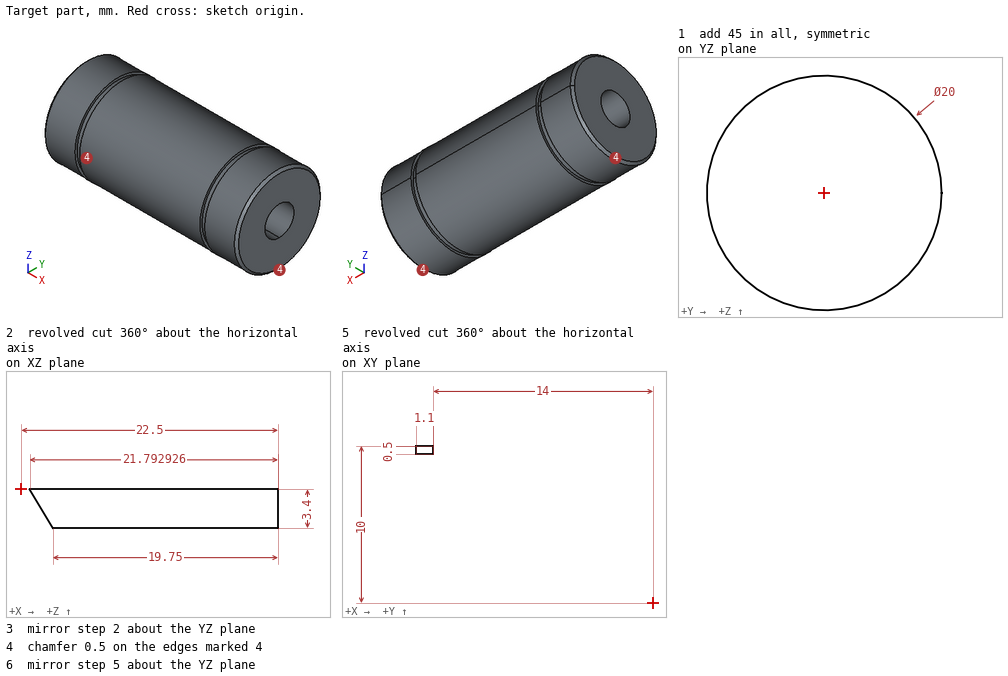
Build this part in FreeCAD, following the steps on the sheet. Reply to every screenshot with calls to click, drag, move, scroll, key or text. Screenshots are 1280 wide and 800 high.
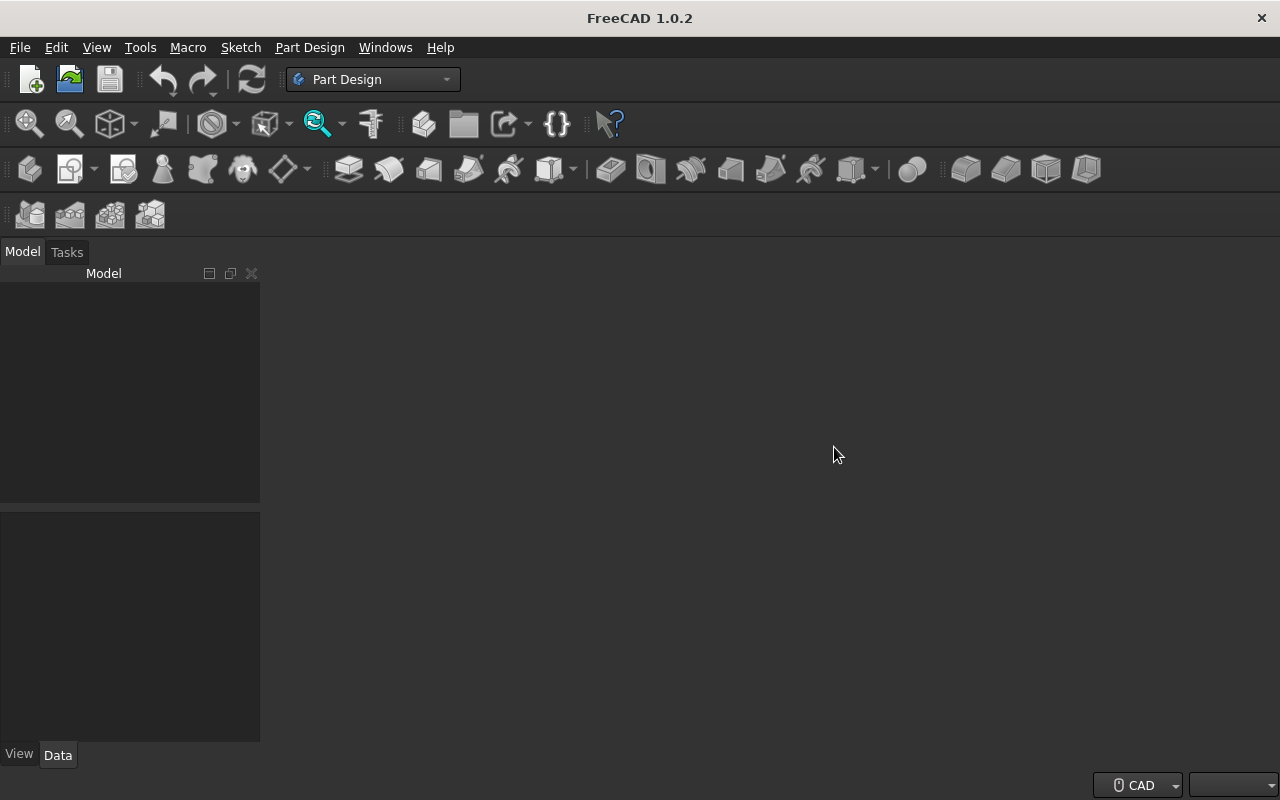
click(30, 80)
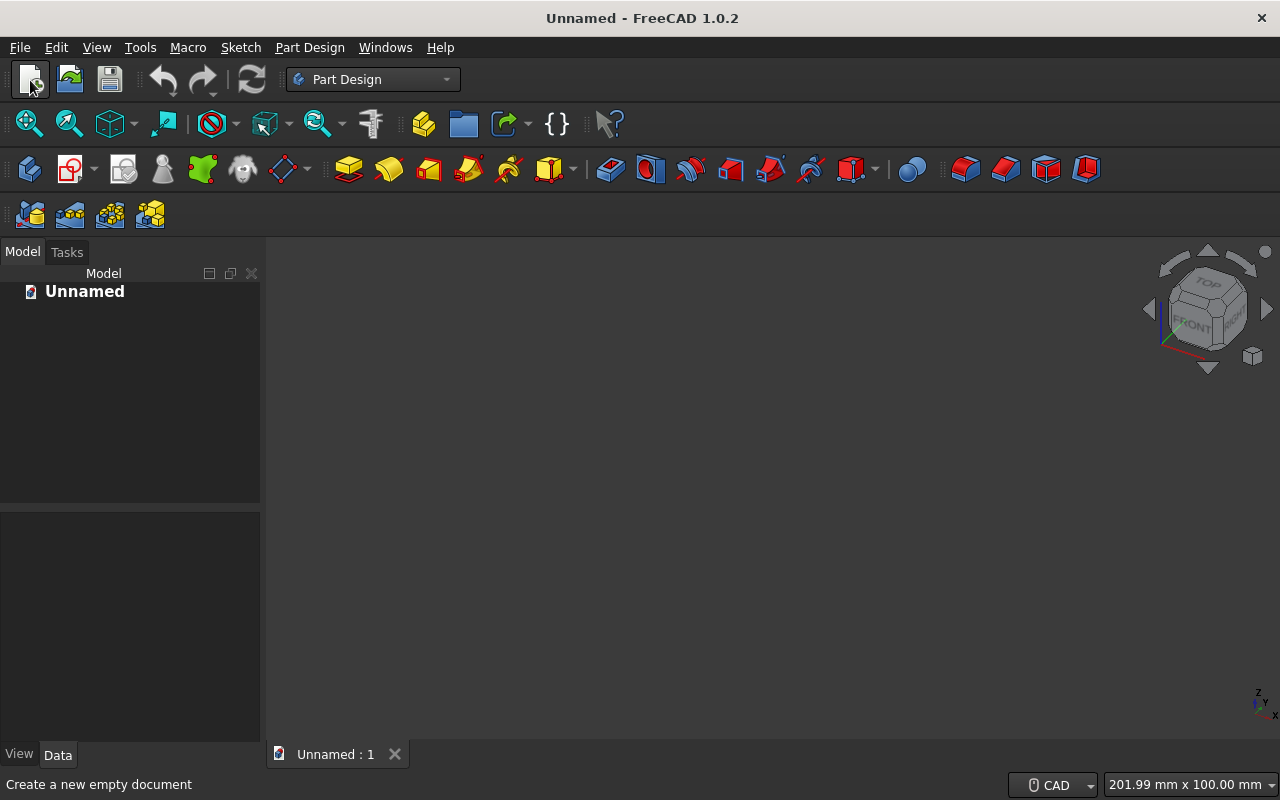
click(70, 170)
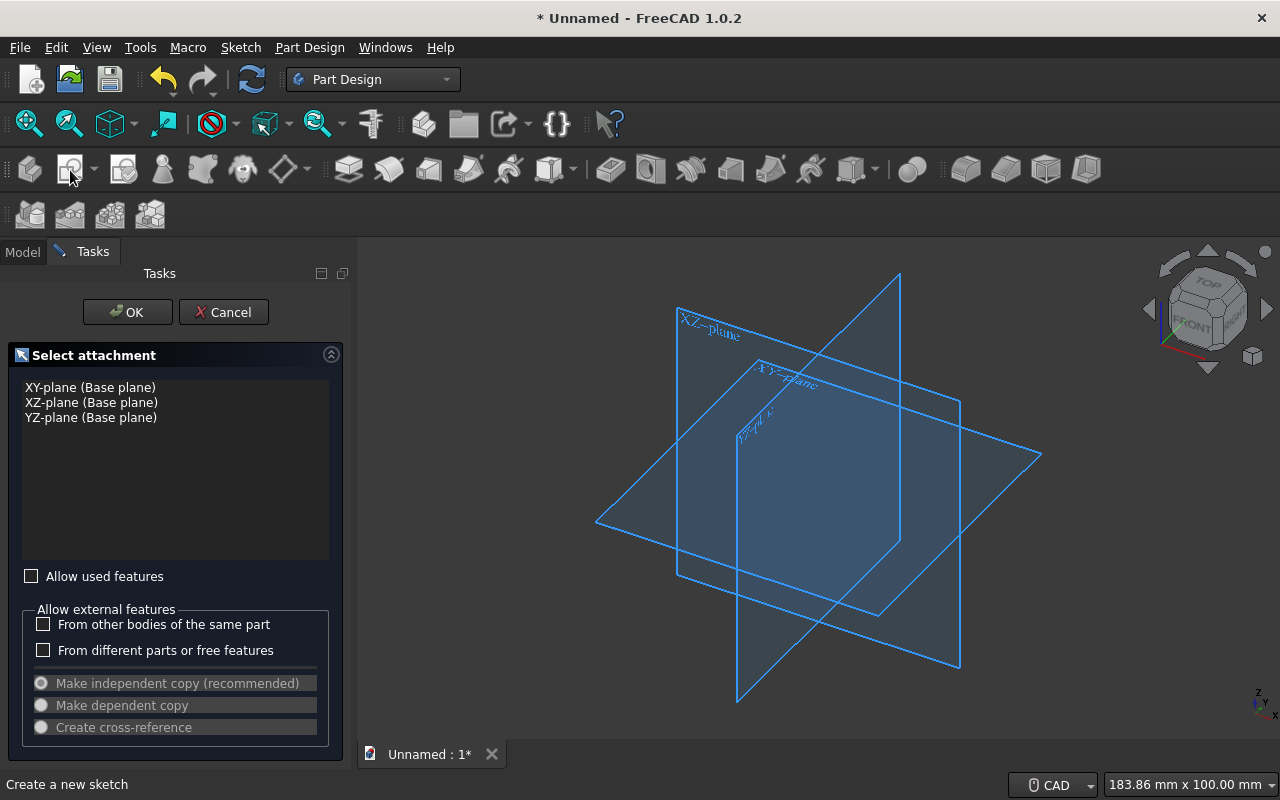
click(82, 418)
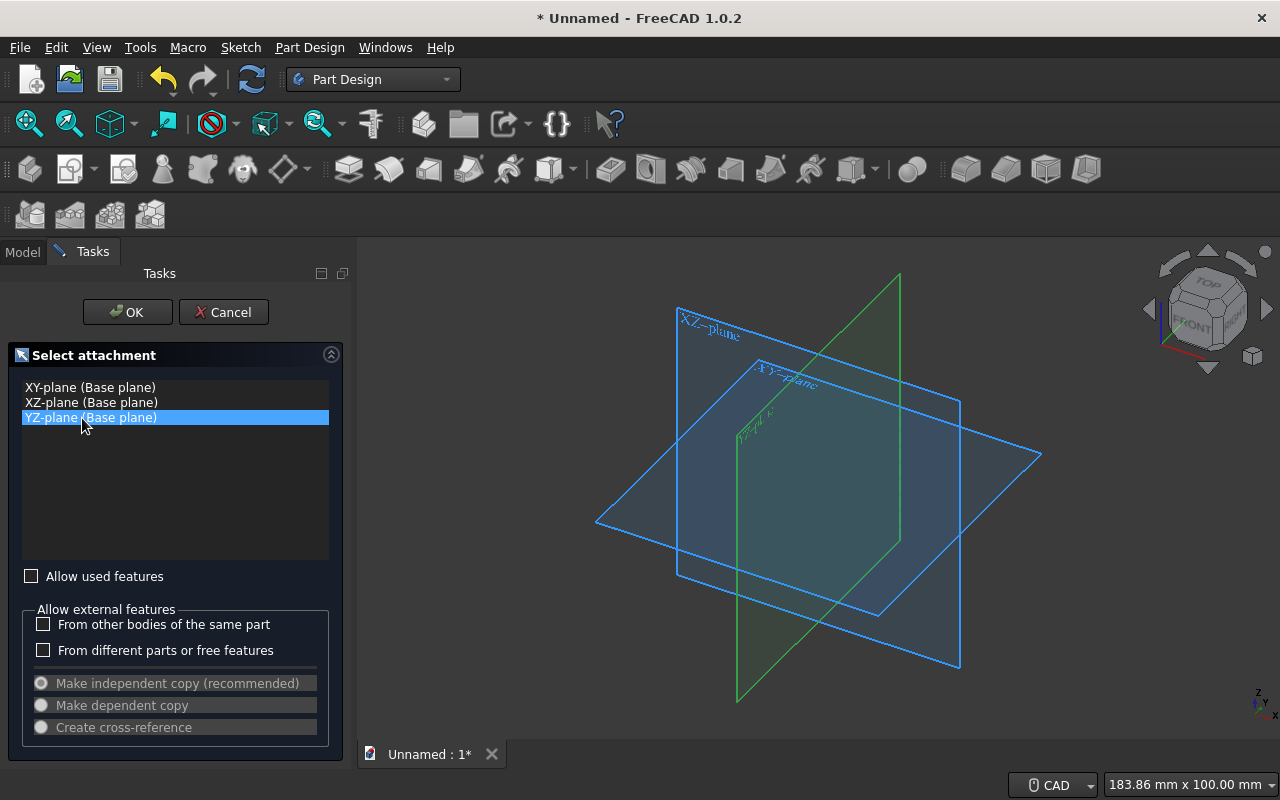
click(128, 312)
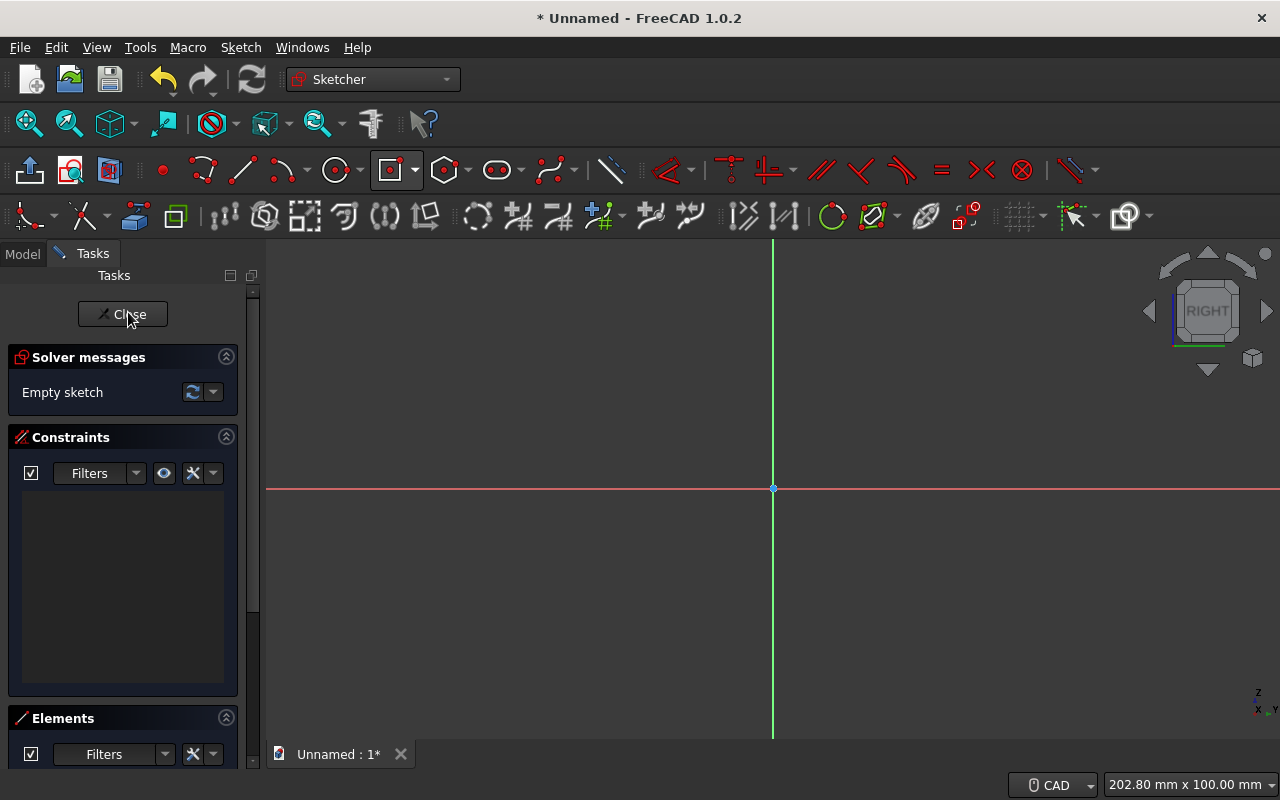
scroll(803, 489, up, 6)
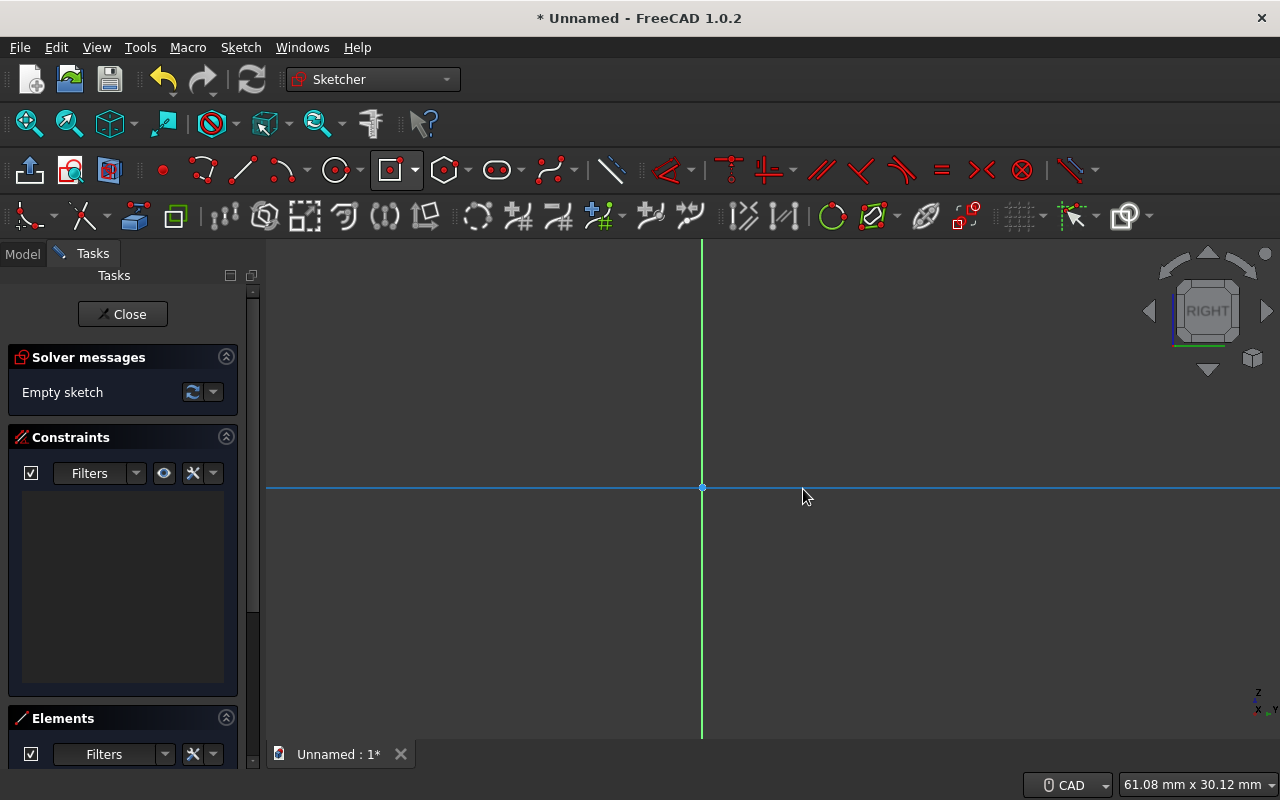
click(336, 170)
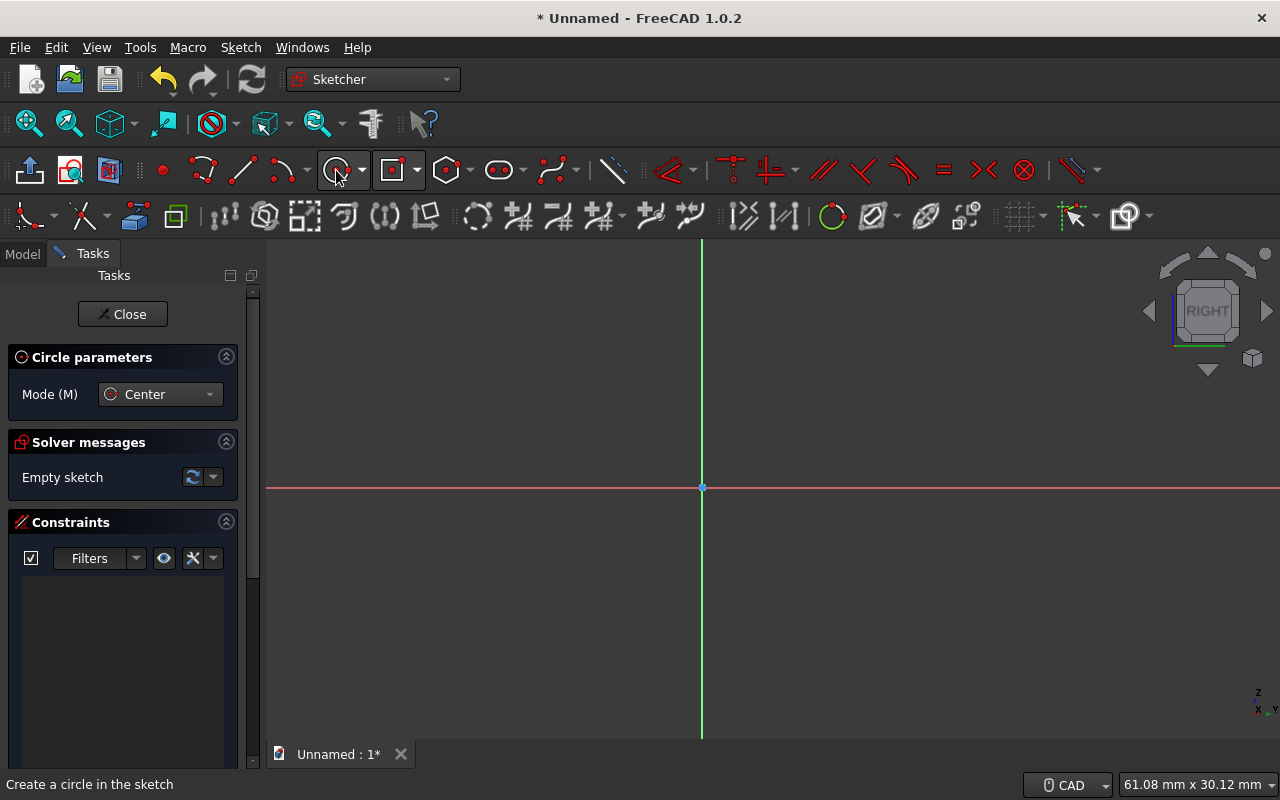
click(702, 488)
move(820, 370)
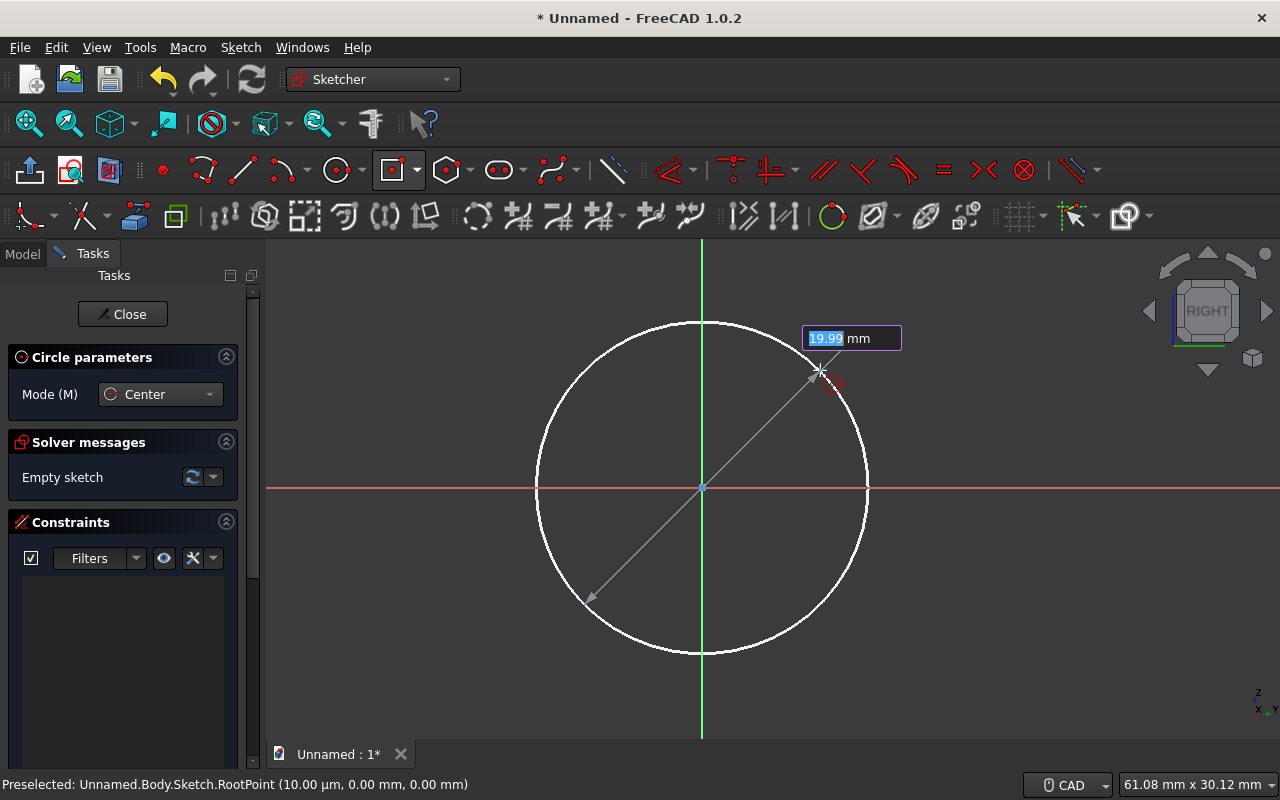
text(20)
key(Return)
key(Escape)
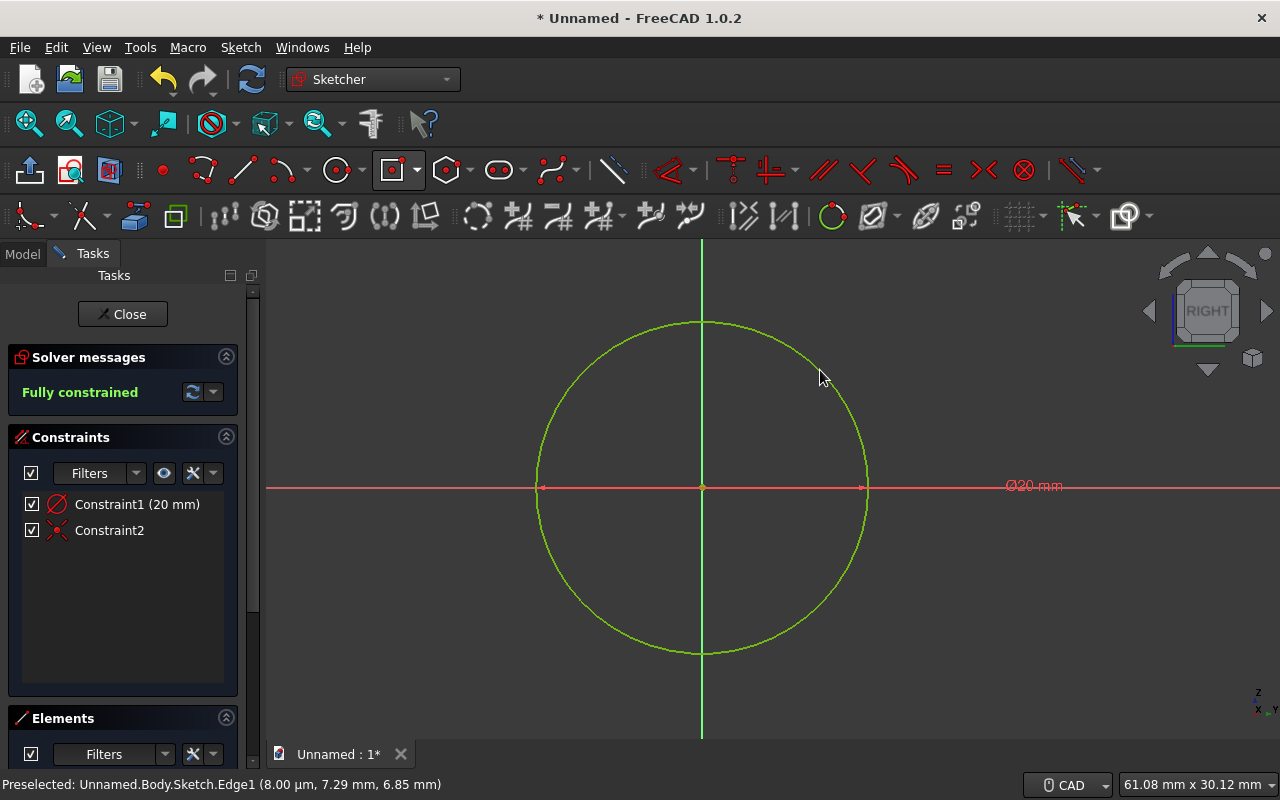
click(123, 314)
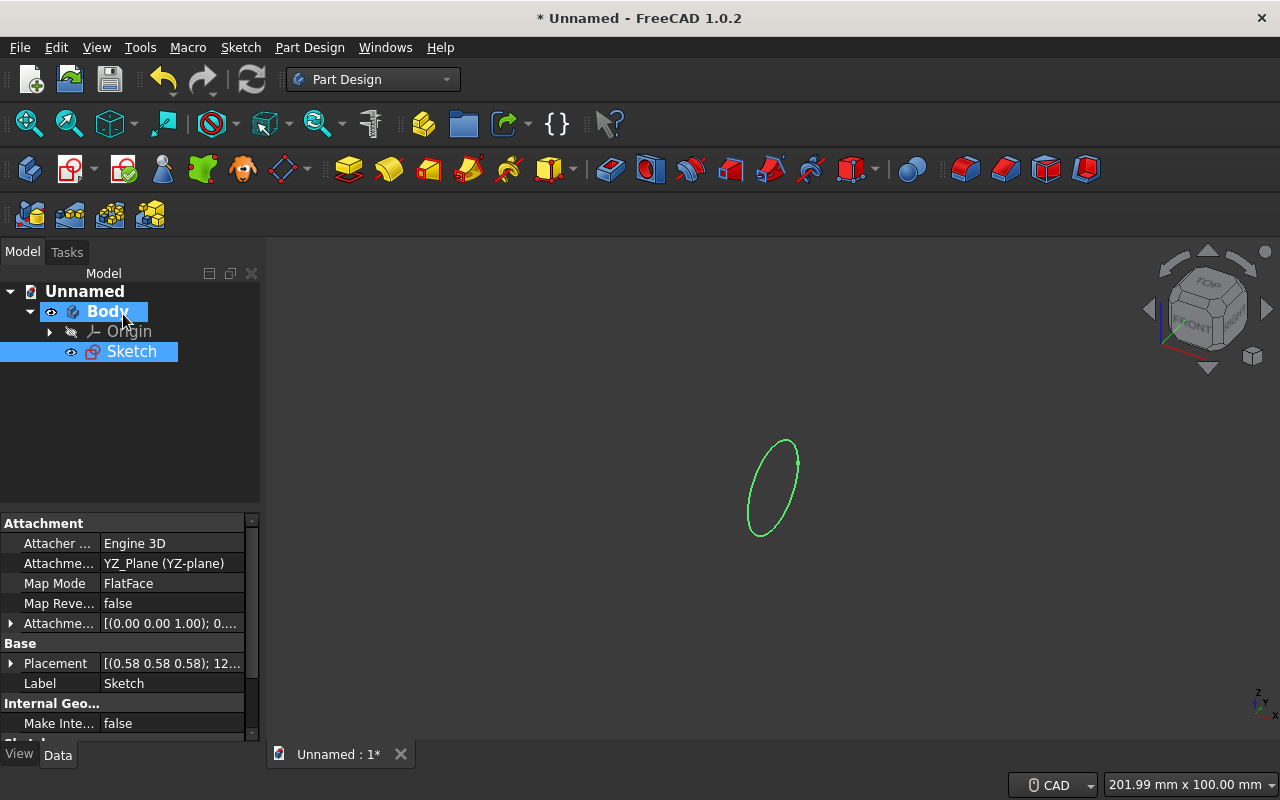
click(350, 170)